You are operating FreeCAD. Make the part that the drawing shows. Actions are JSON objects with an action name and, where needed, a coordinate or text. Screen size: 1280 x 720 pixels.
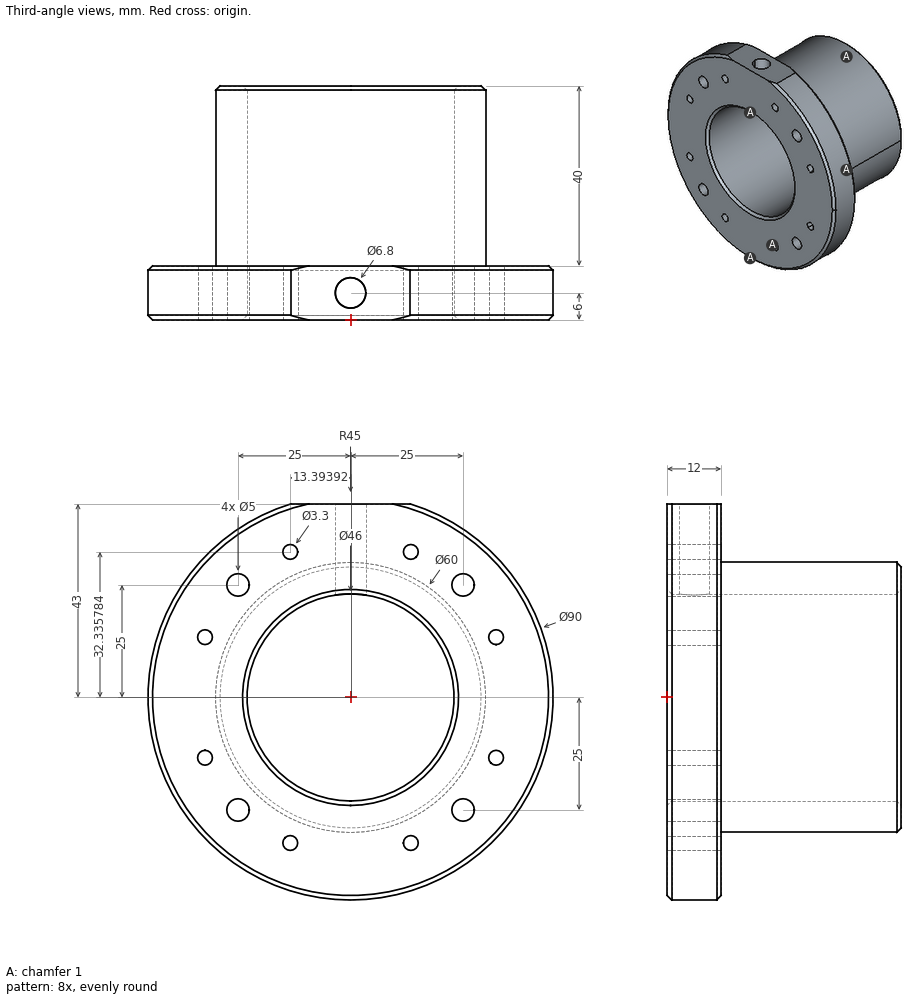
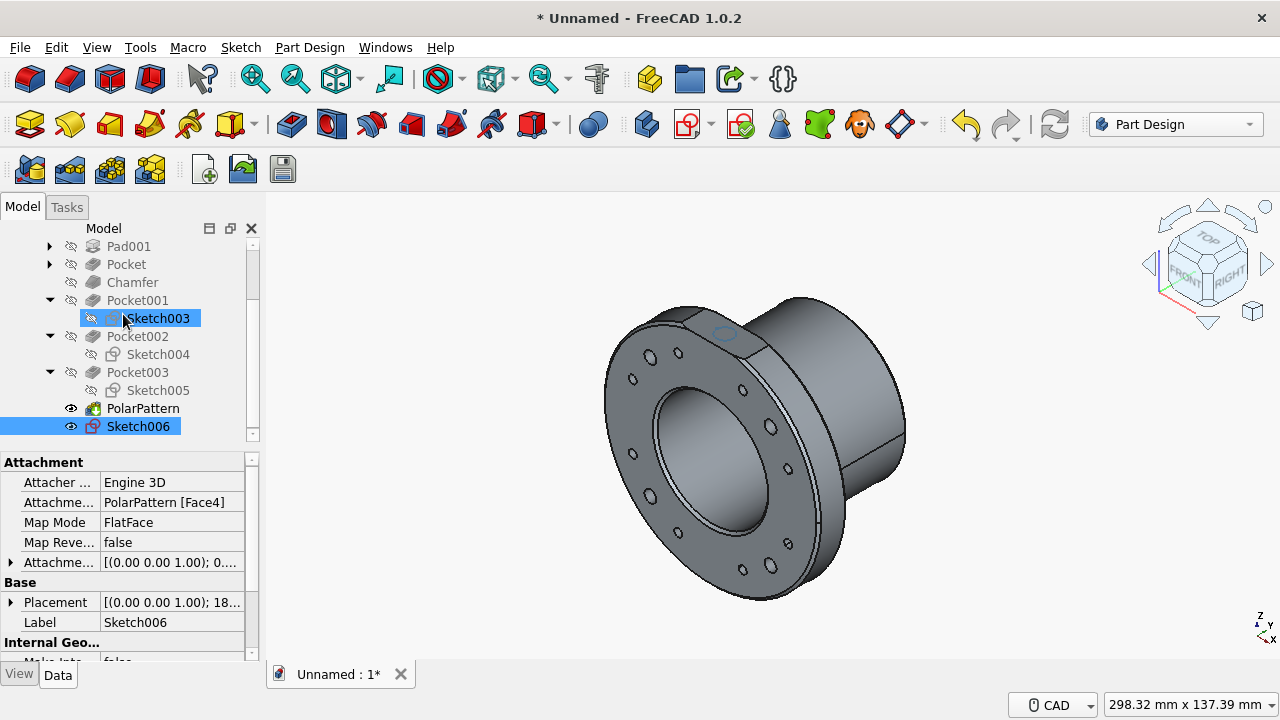
{"action": "left_click", "coordinate": [292, 124]}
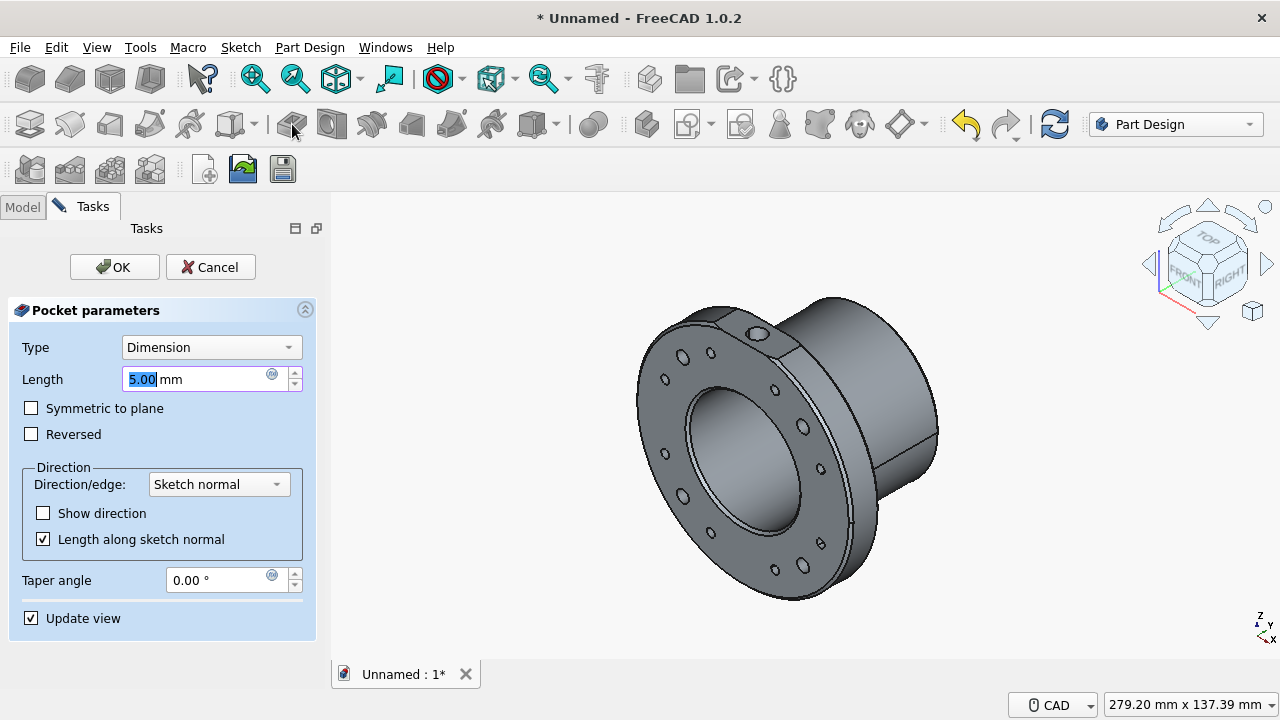
{"action": "left_click", "coordinate": [212, 348]}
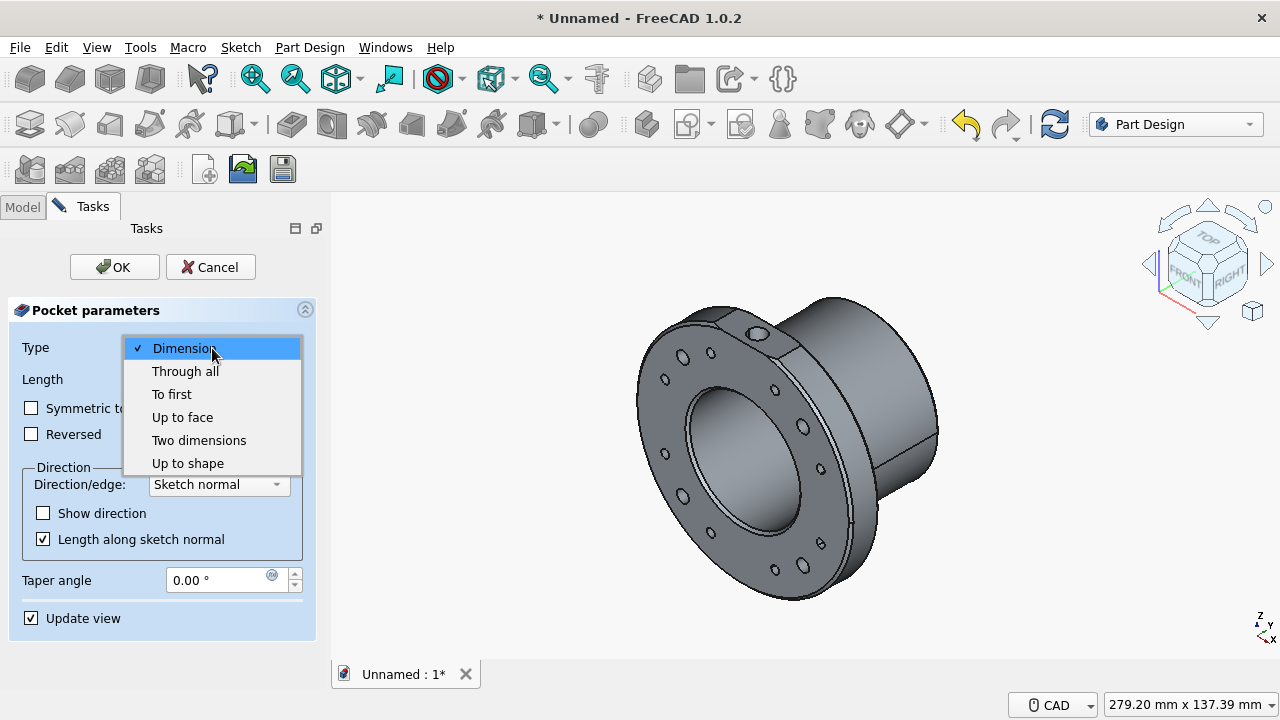
{"action": "left_click", "coordinate": [212, 394]}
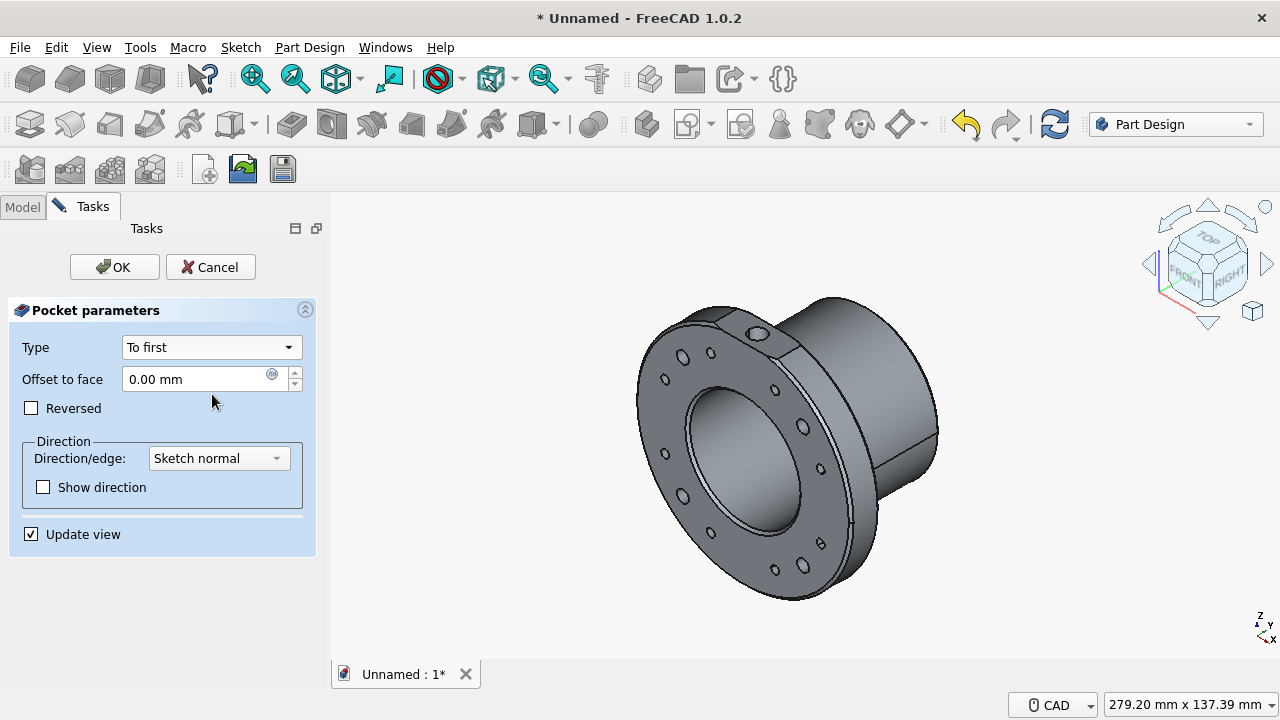
{"action": "left_click", "coordinate": [115, 267]}